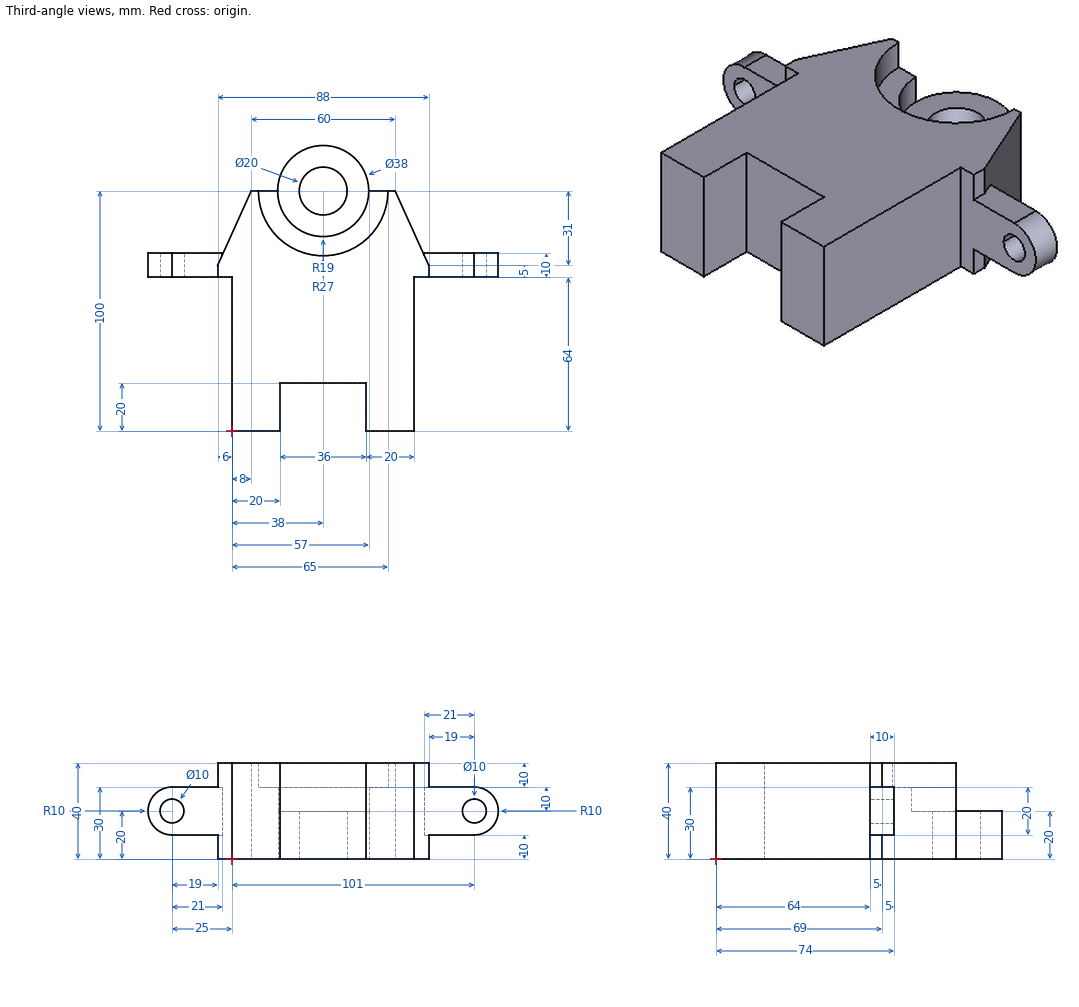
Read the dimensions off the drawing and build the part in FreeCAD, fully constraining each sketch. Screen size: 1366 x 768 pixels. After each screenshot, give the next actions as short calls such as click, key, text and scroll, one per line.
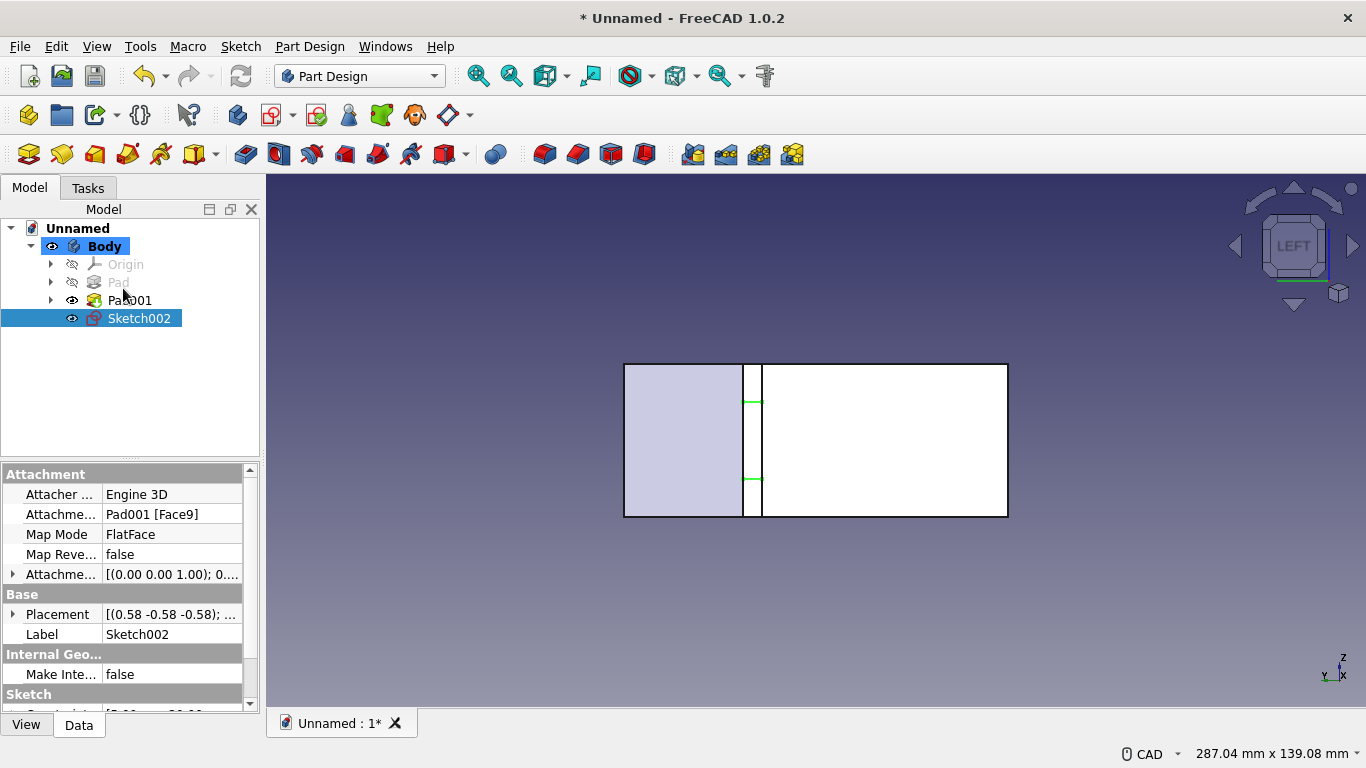
click(29, 154)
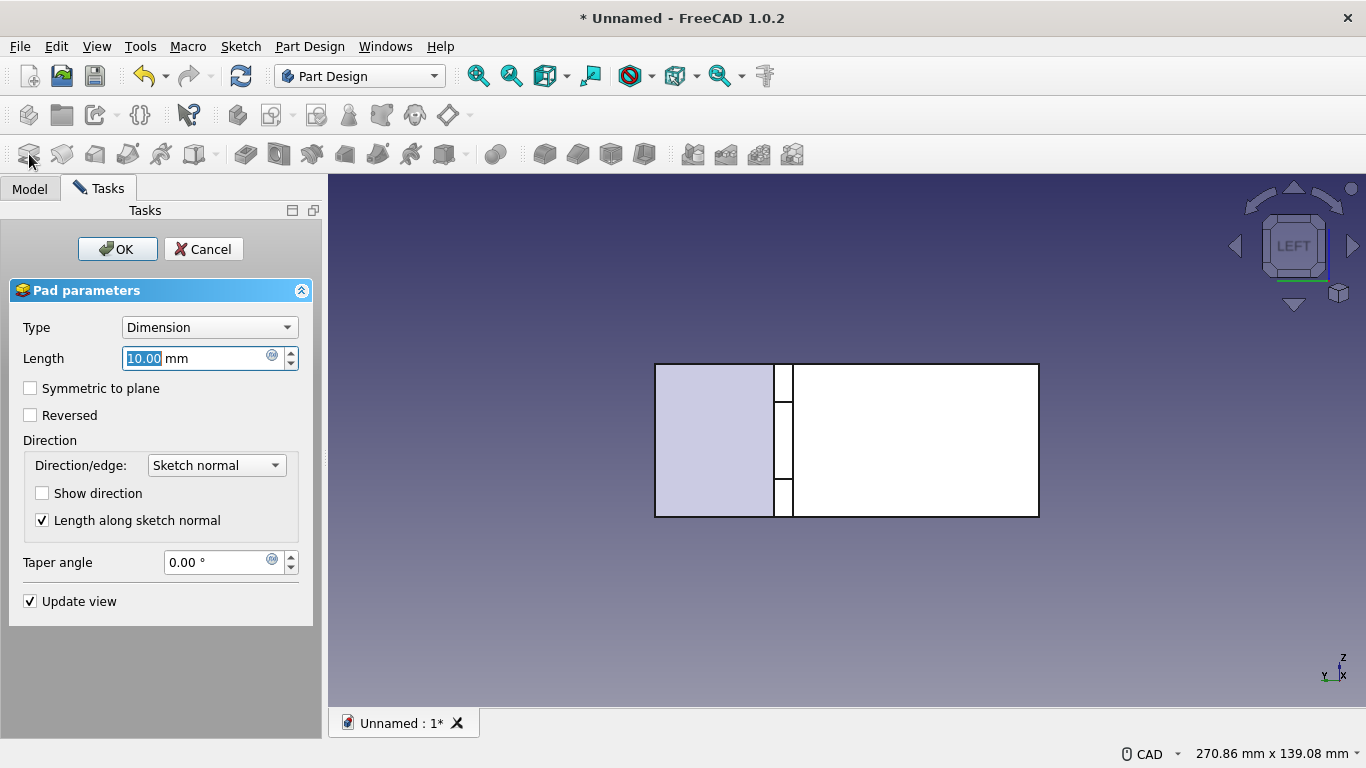
text(19)
key(Tab)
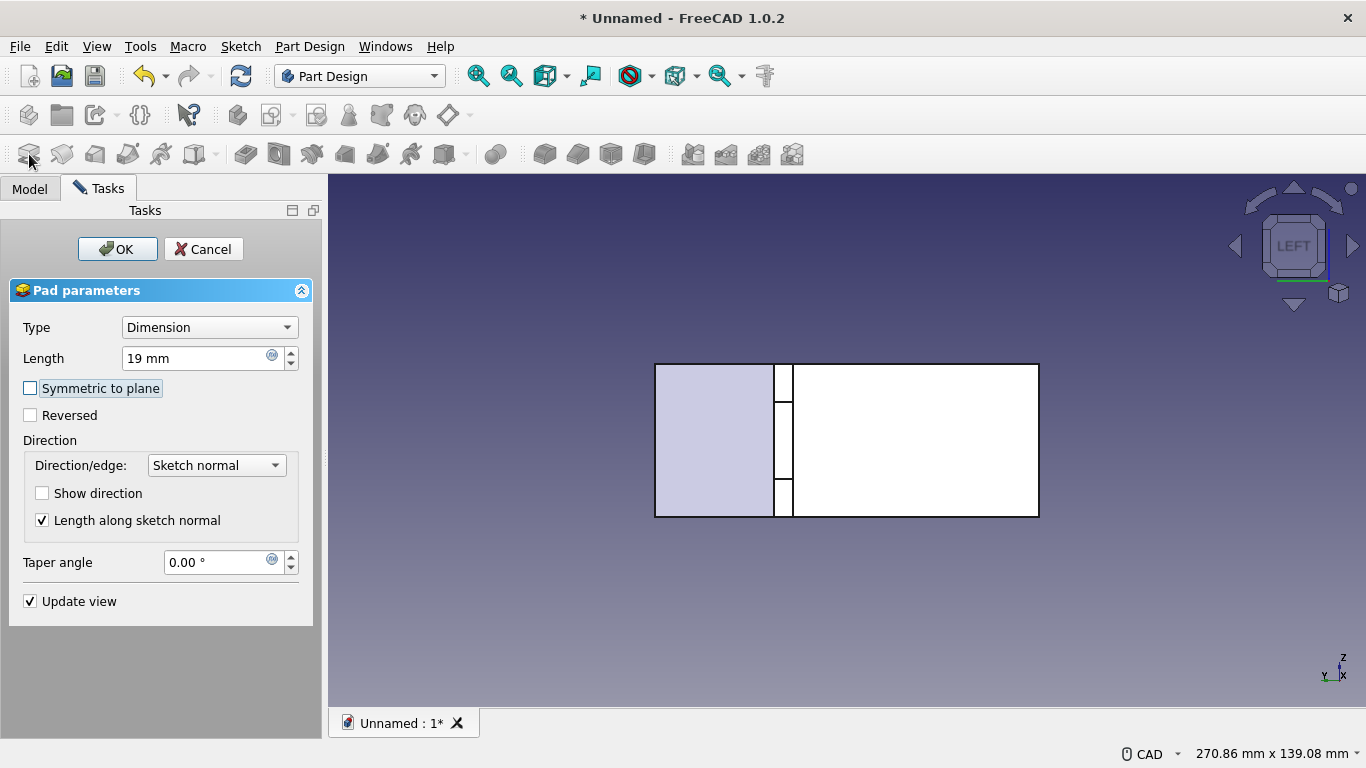
click(118, 249)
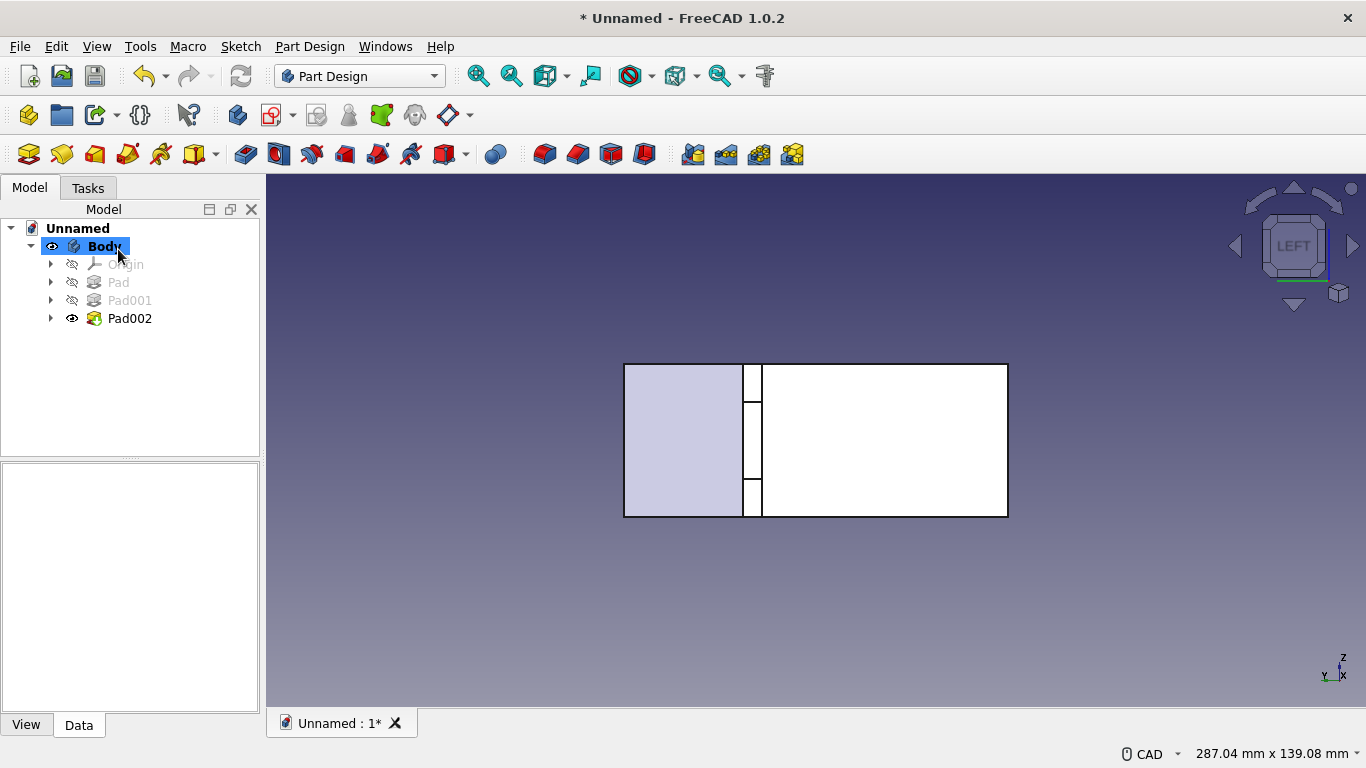
click(479, 76)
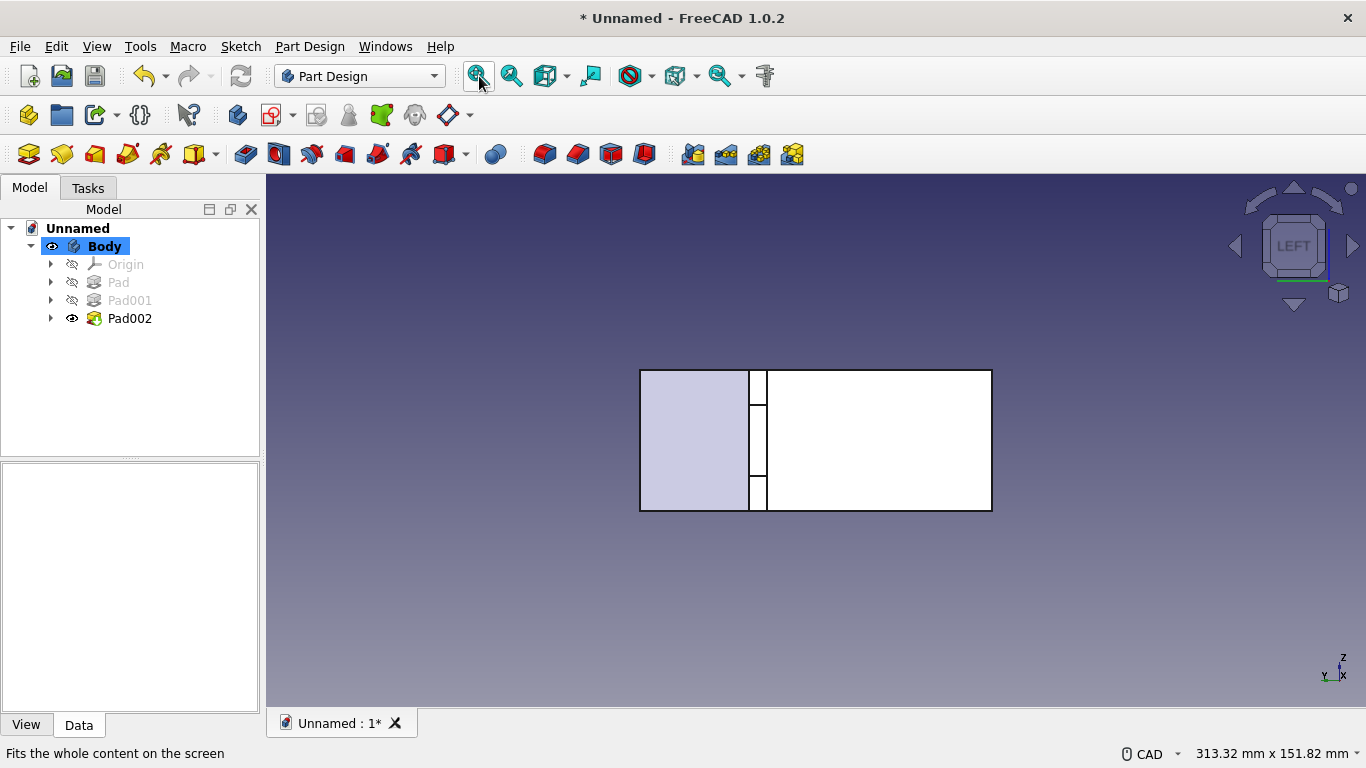
click(758, 419)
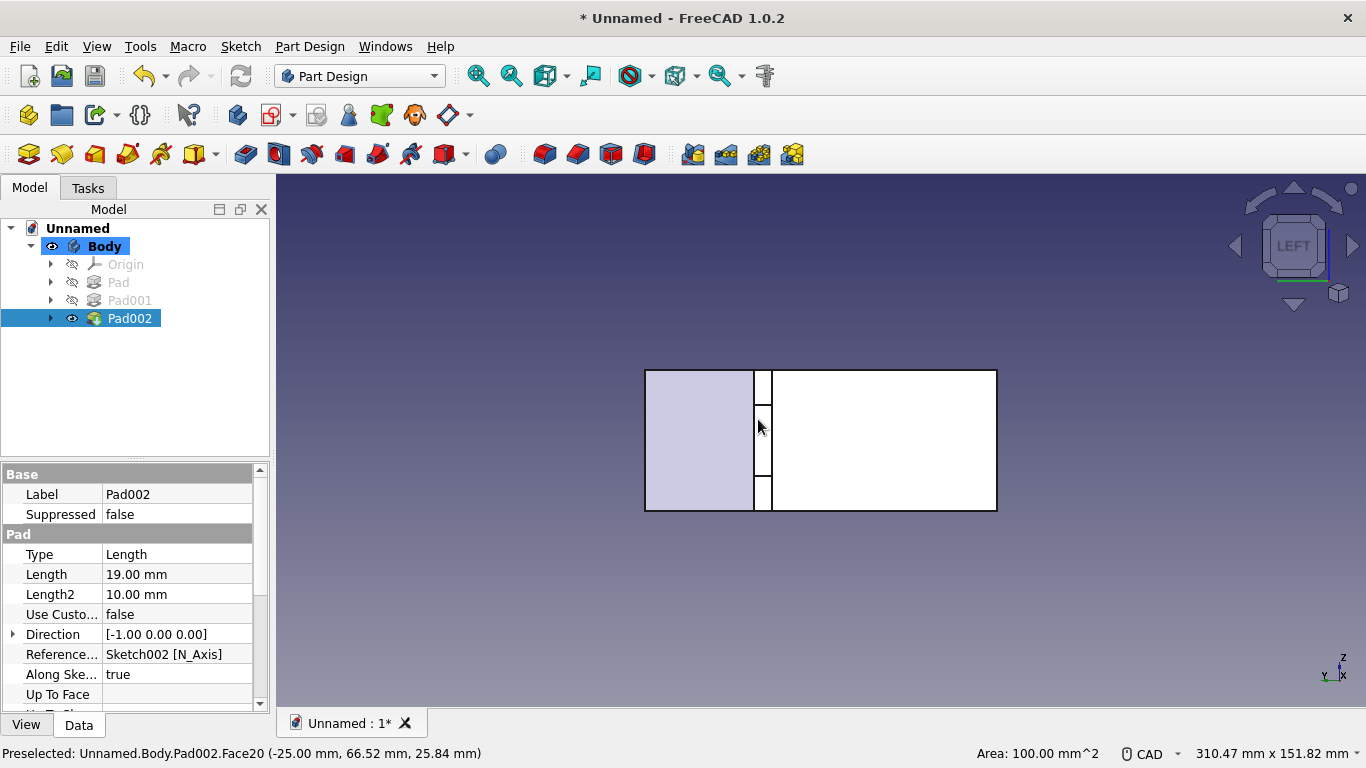
click(270, 116)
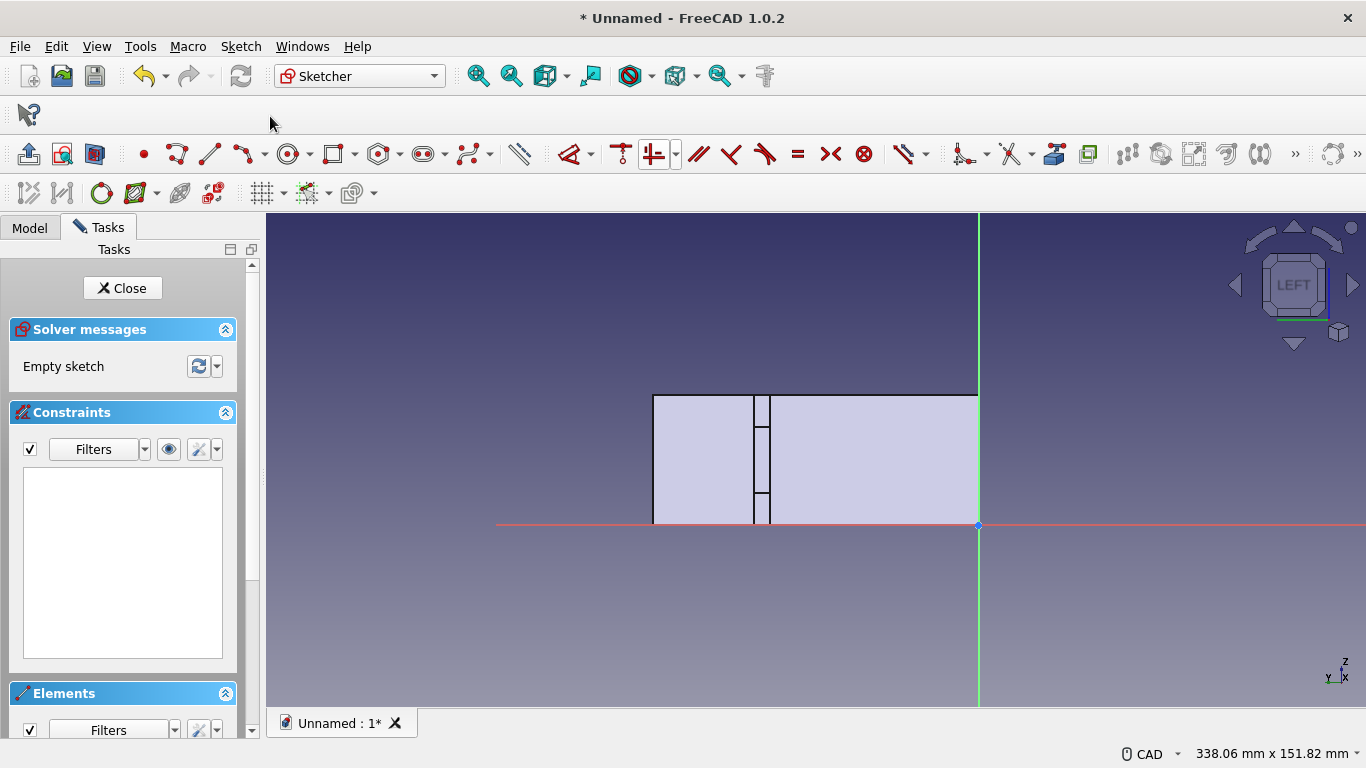
scroll(746, 460, up, 8)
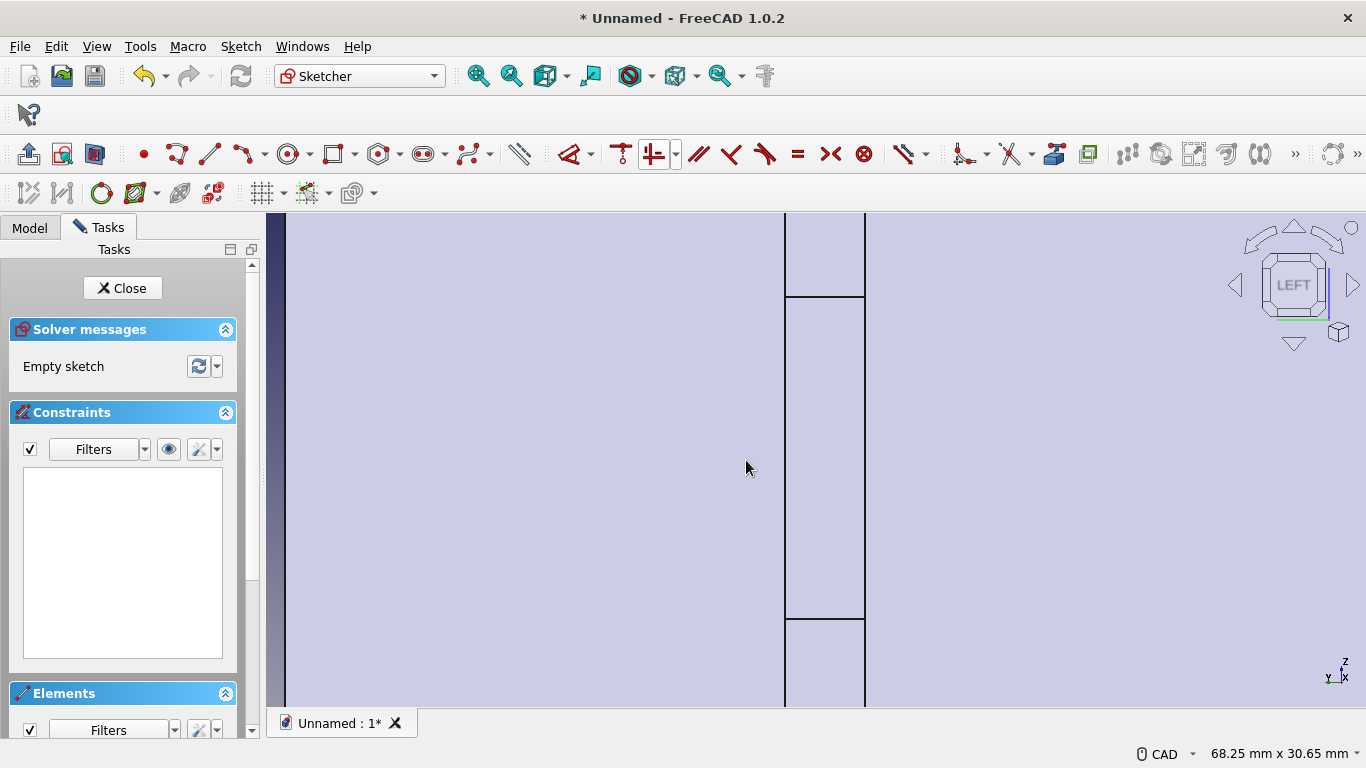
click(332, 154)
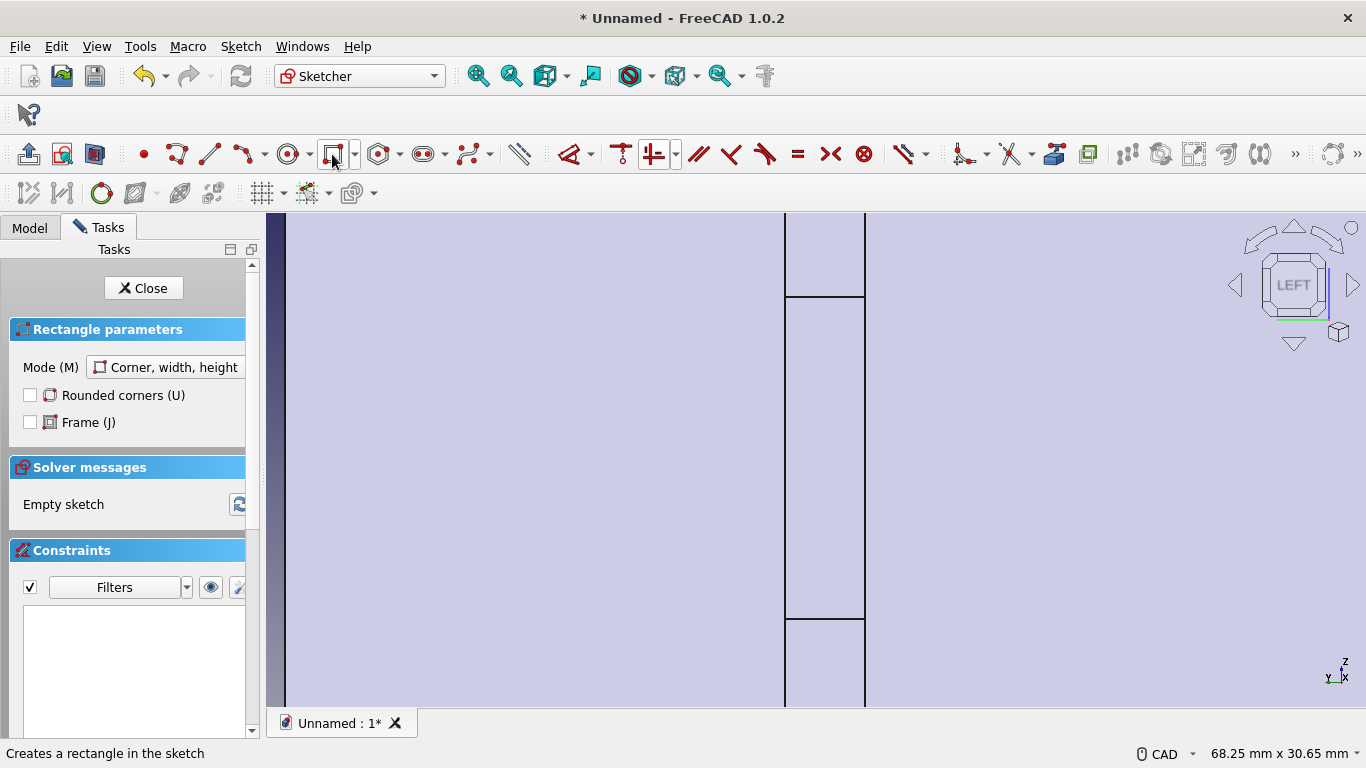
click(704, 297)
click(785, 619)
key(Escape)